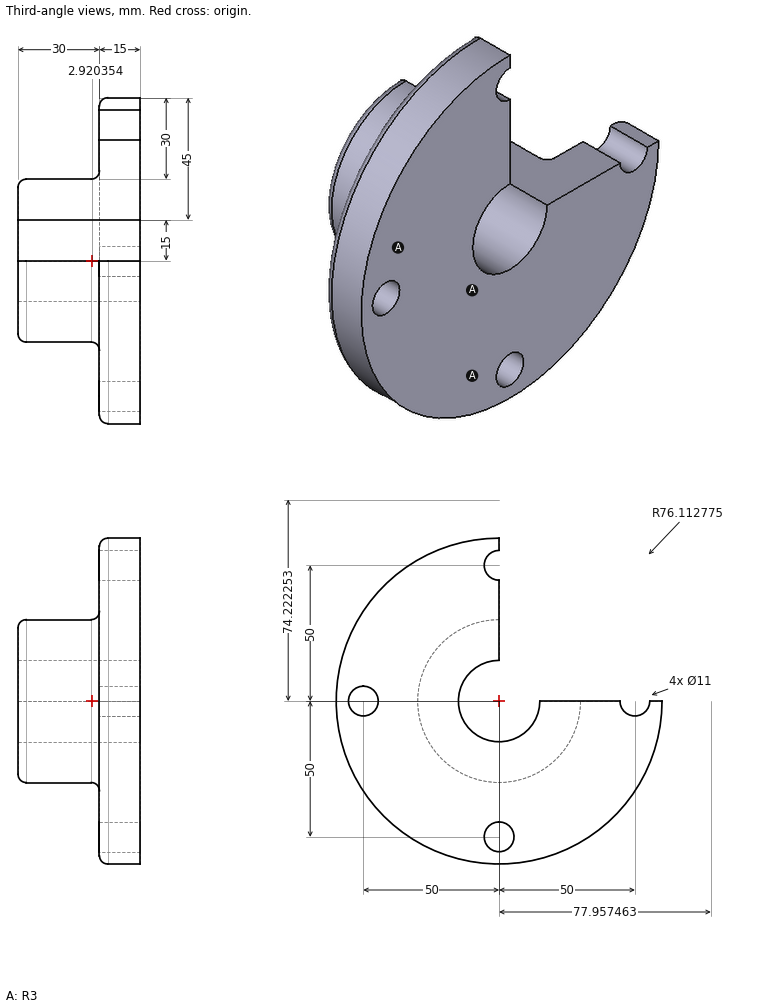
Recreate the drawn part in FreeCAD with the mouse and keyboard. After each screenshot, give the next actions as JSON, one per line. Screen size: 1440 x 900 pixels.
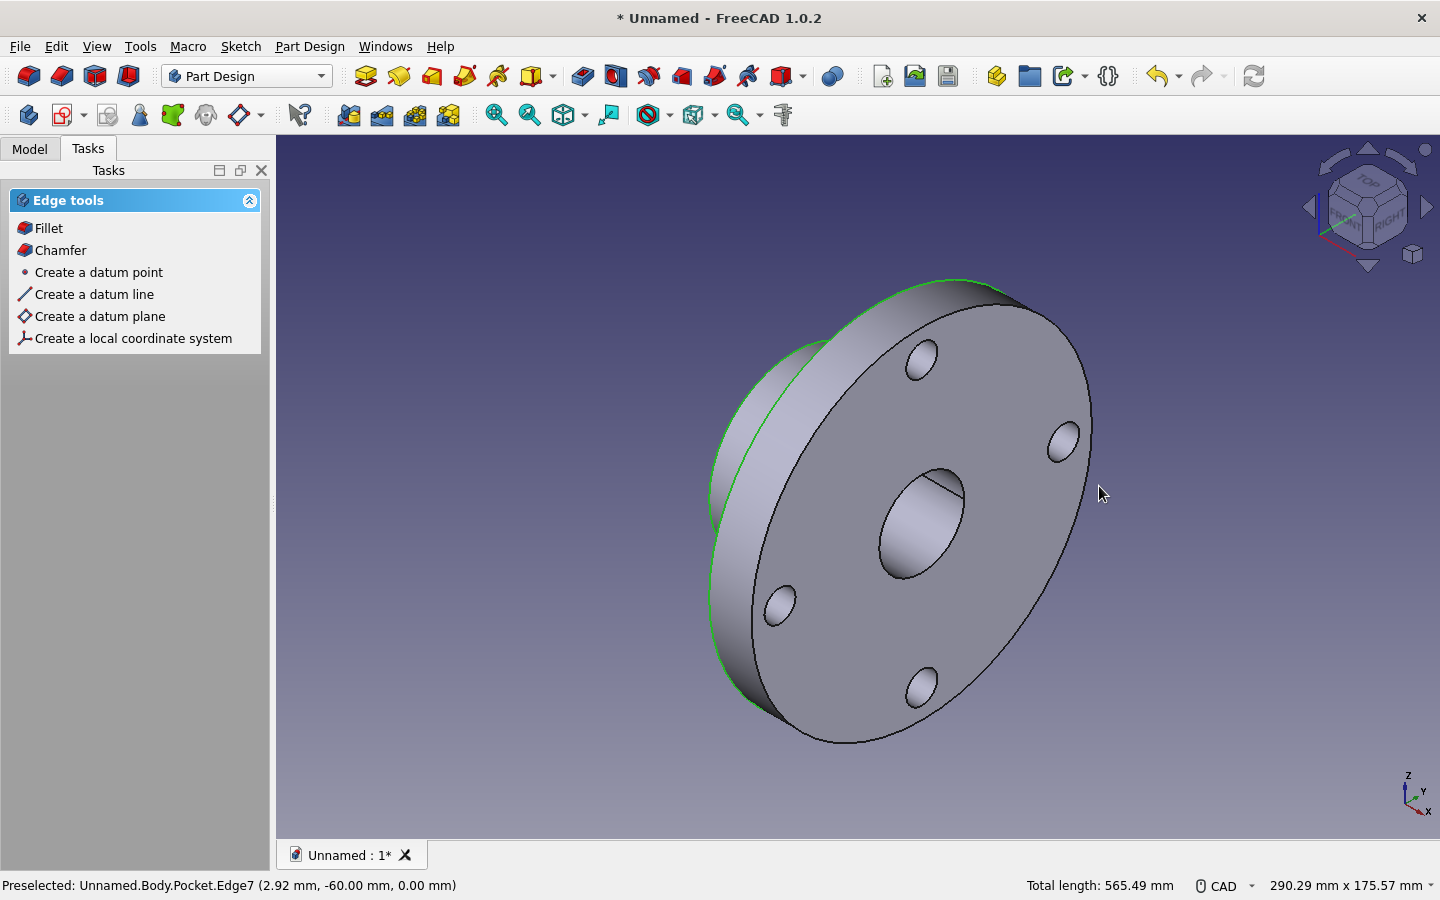
{"action": "key", "text": "2"}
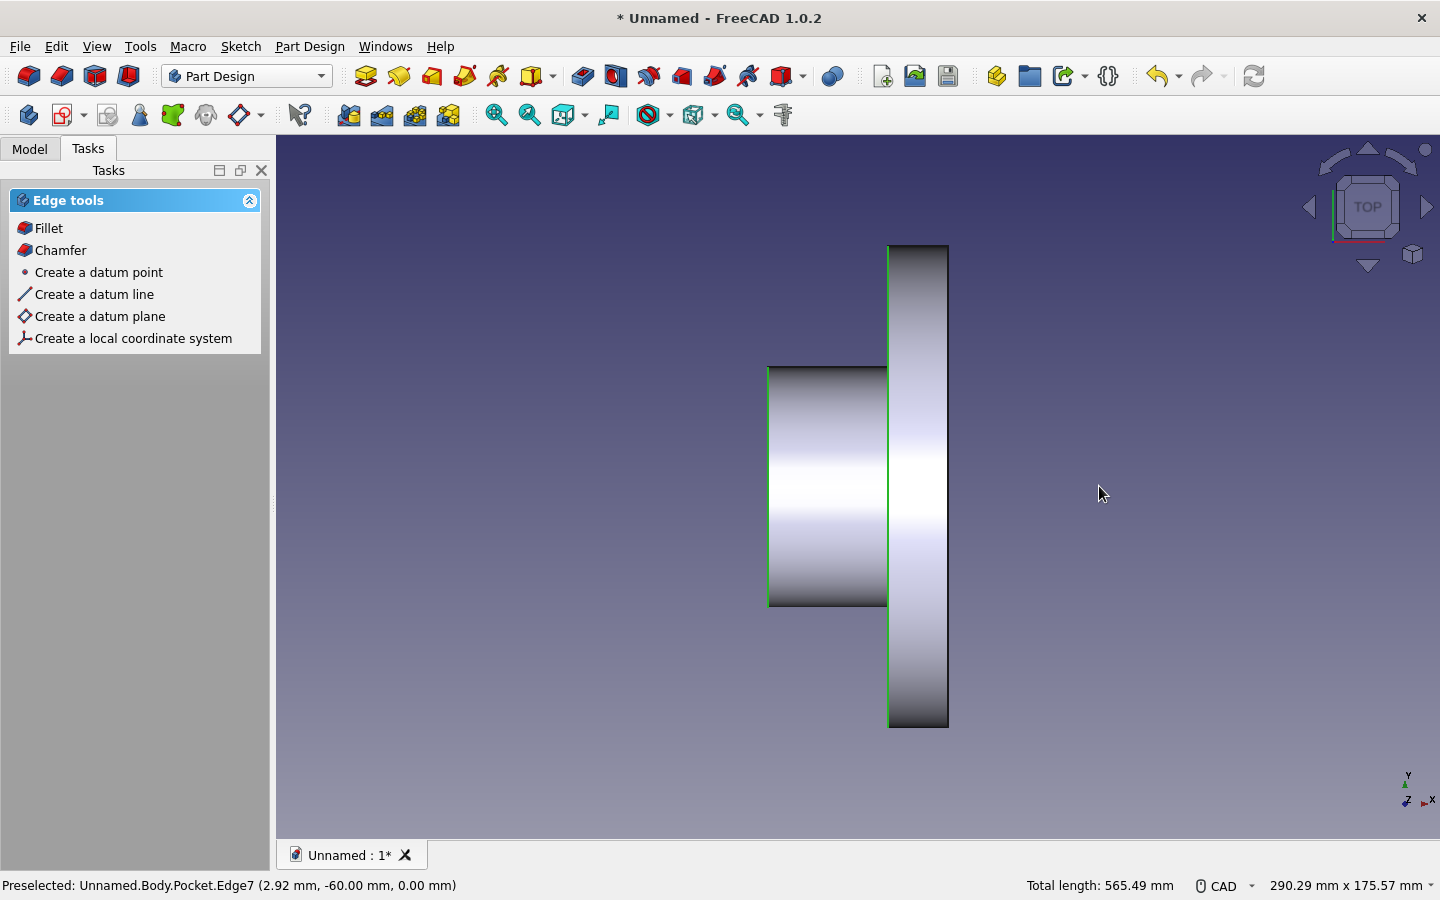
{"action": "key", "text": "1"}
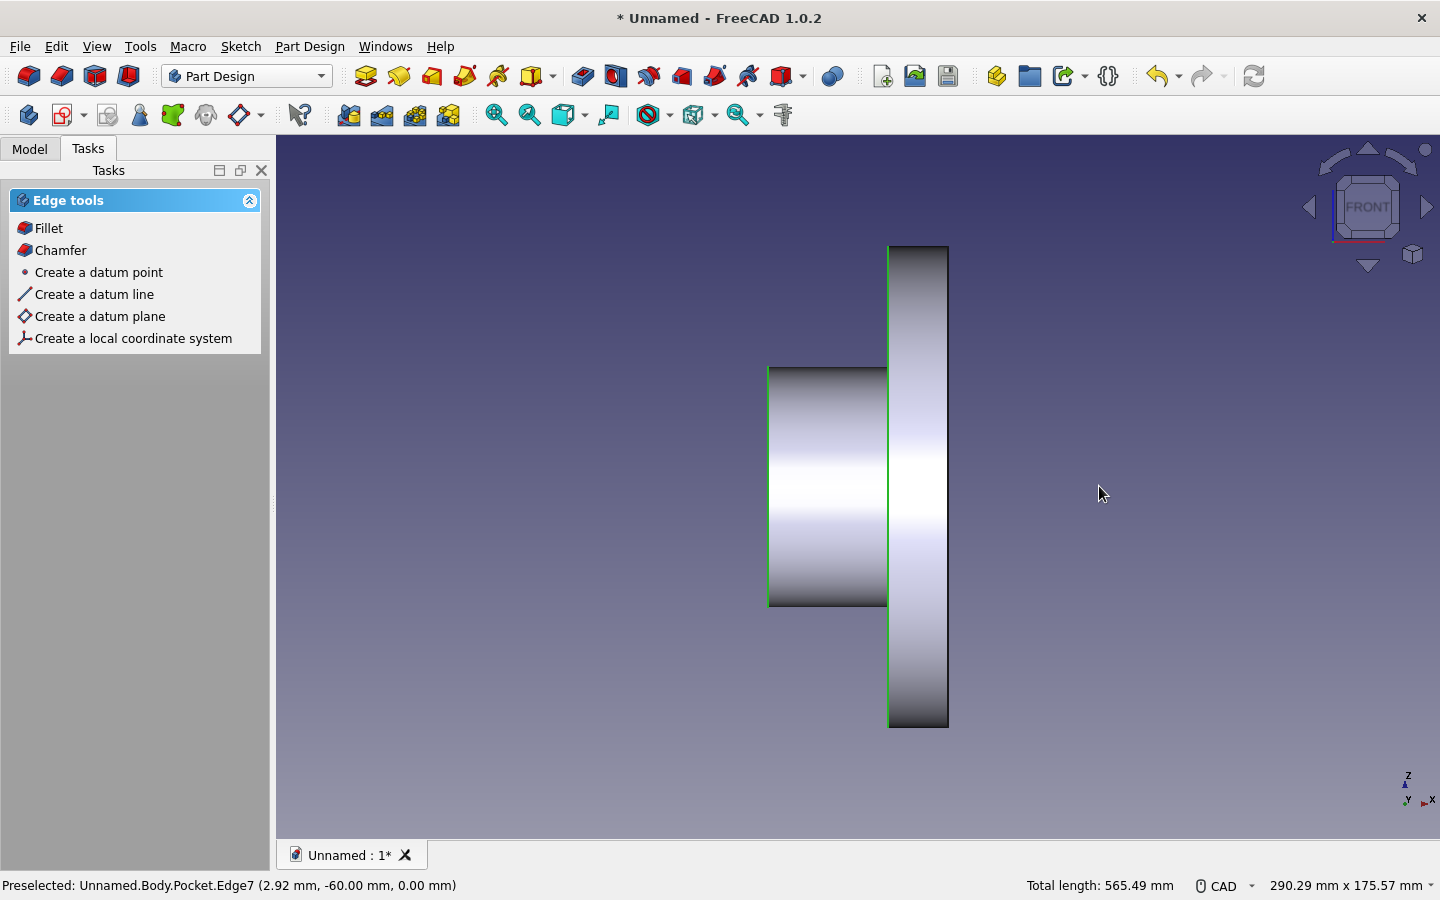
{"action": "key", "text": "3"}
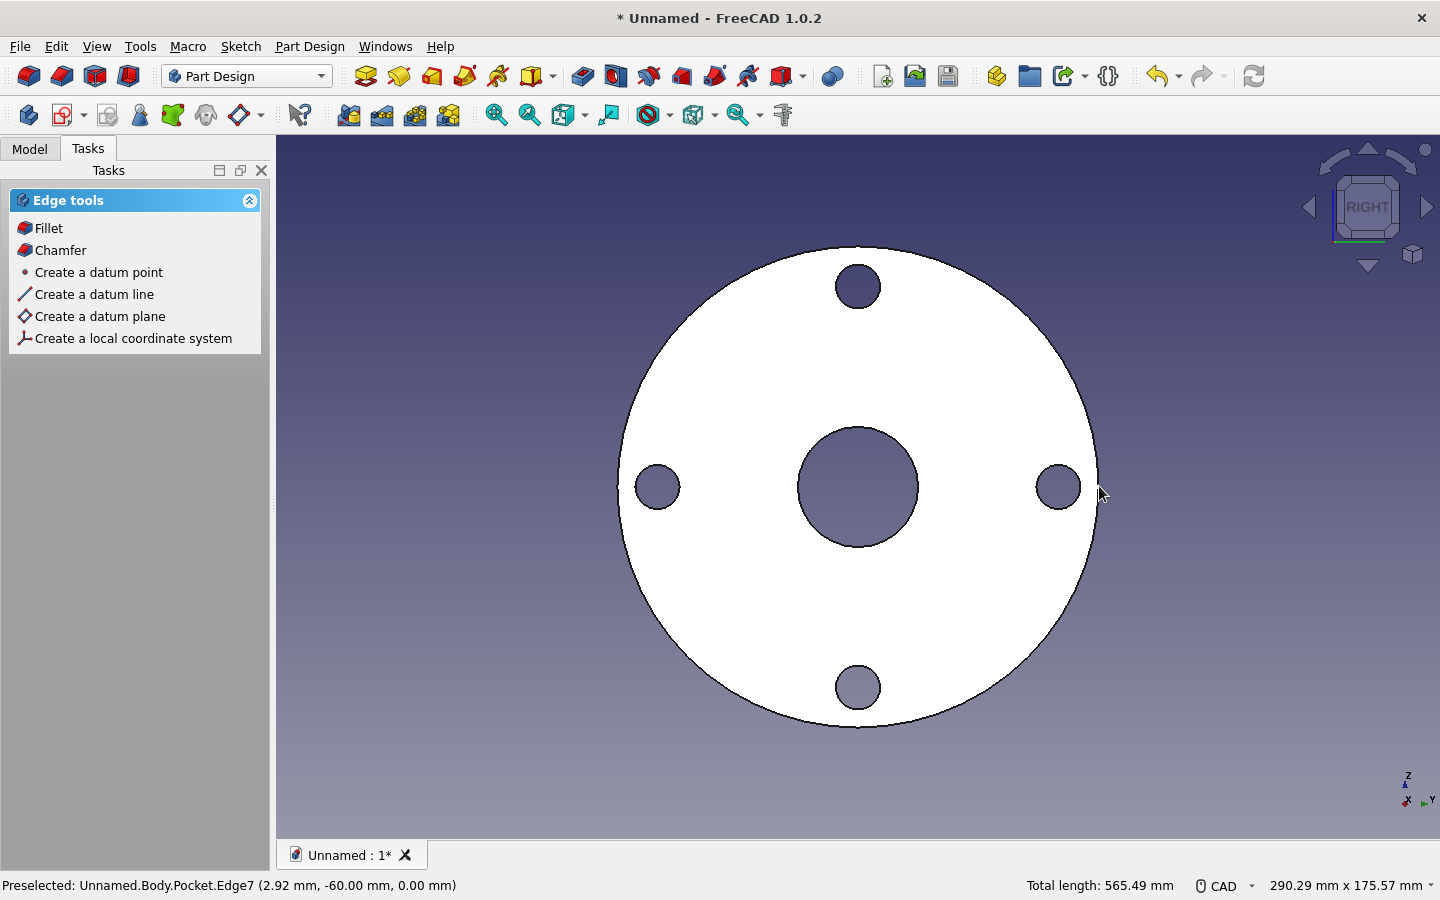
{"action": "key", "text": "5"}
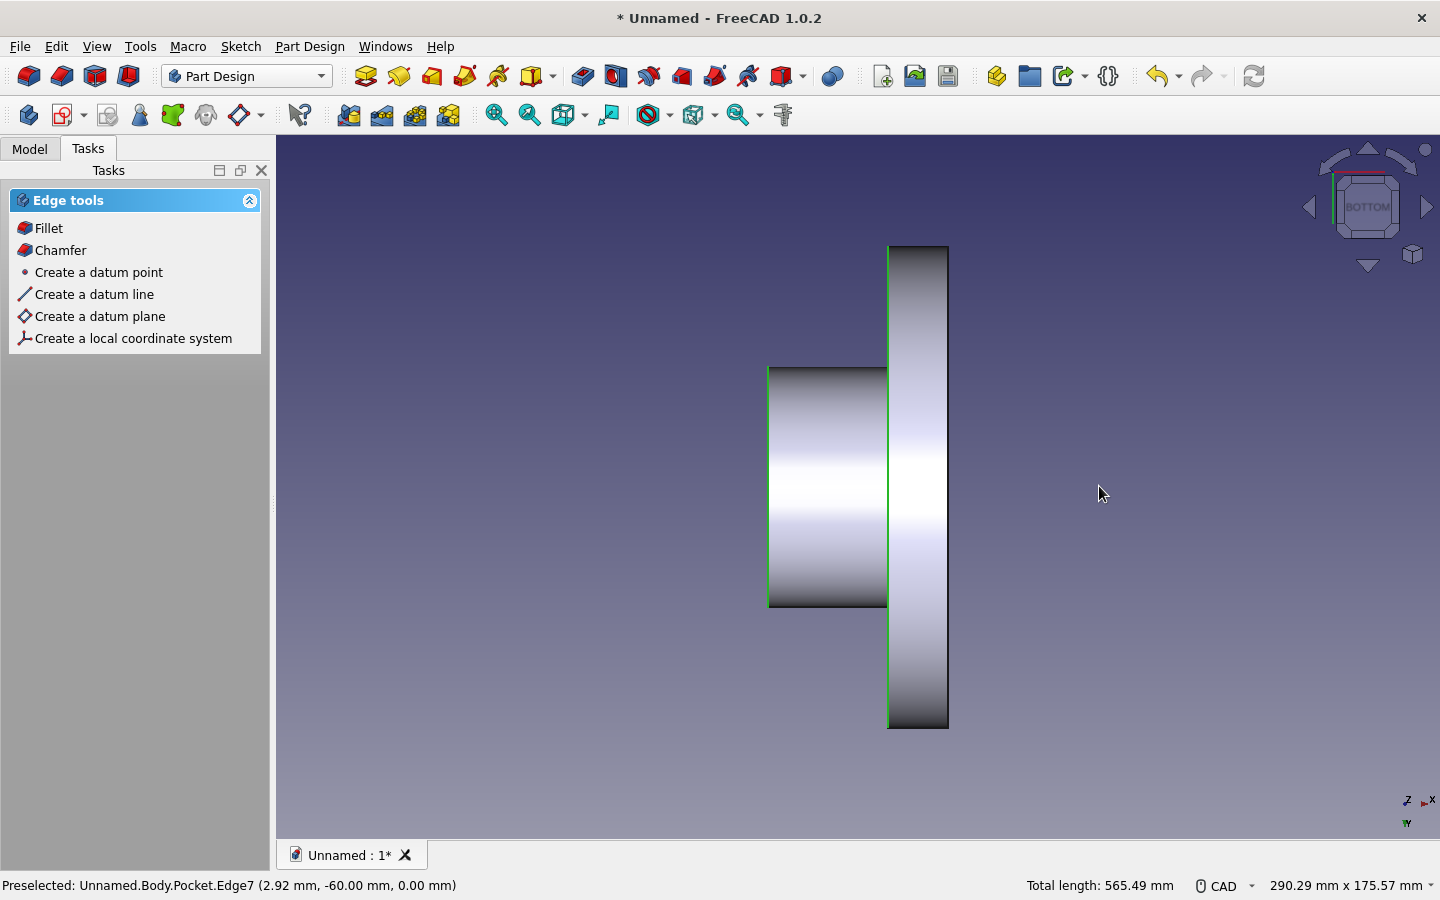
{"action": "key", "text": "4"}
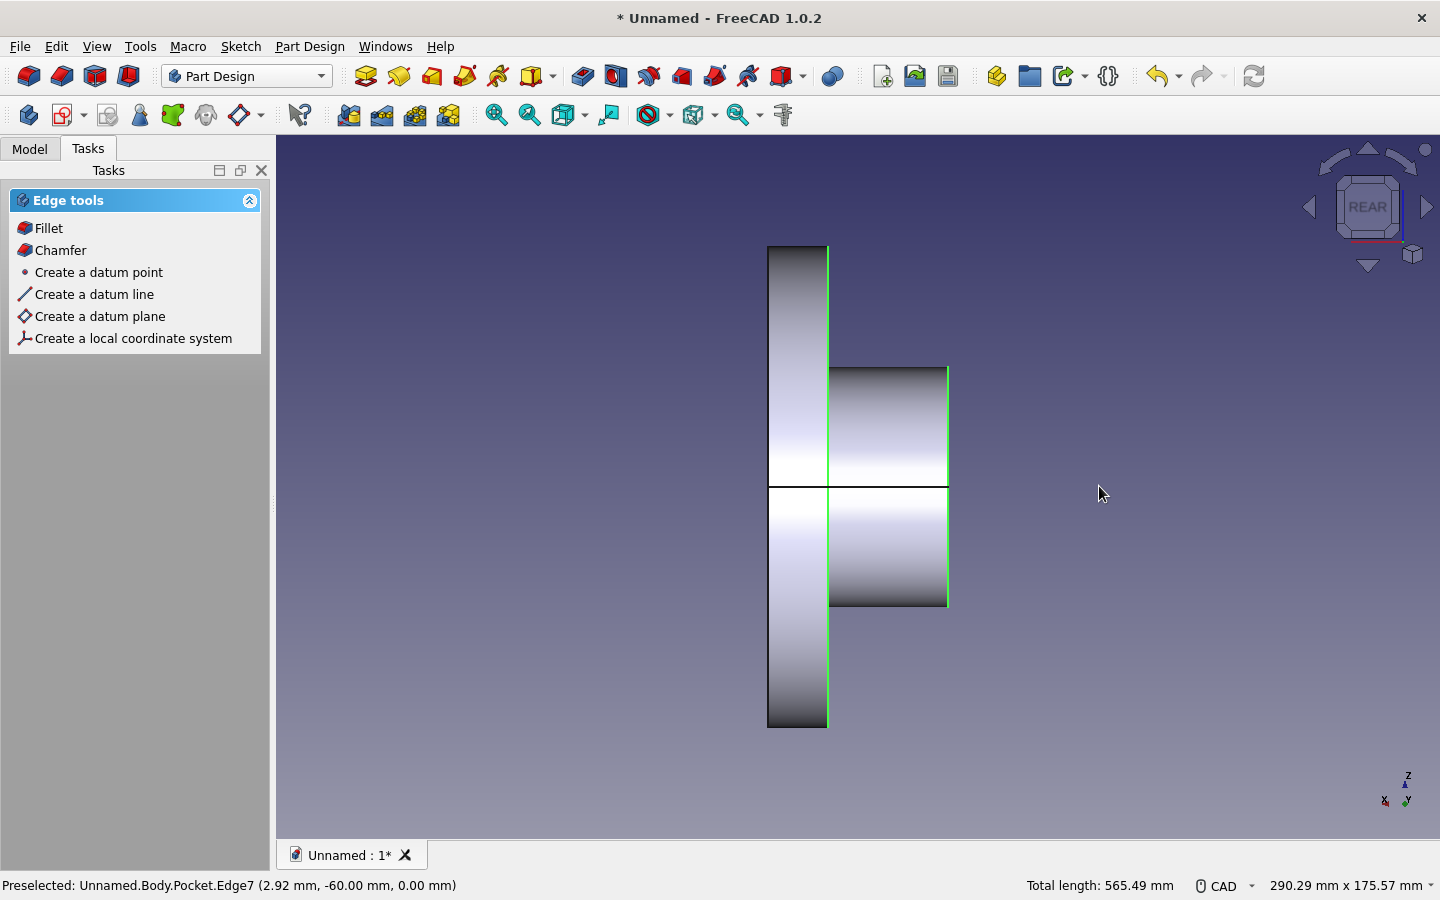
{"action": "key", "text": "6"}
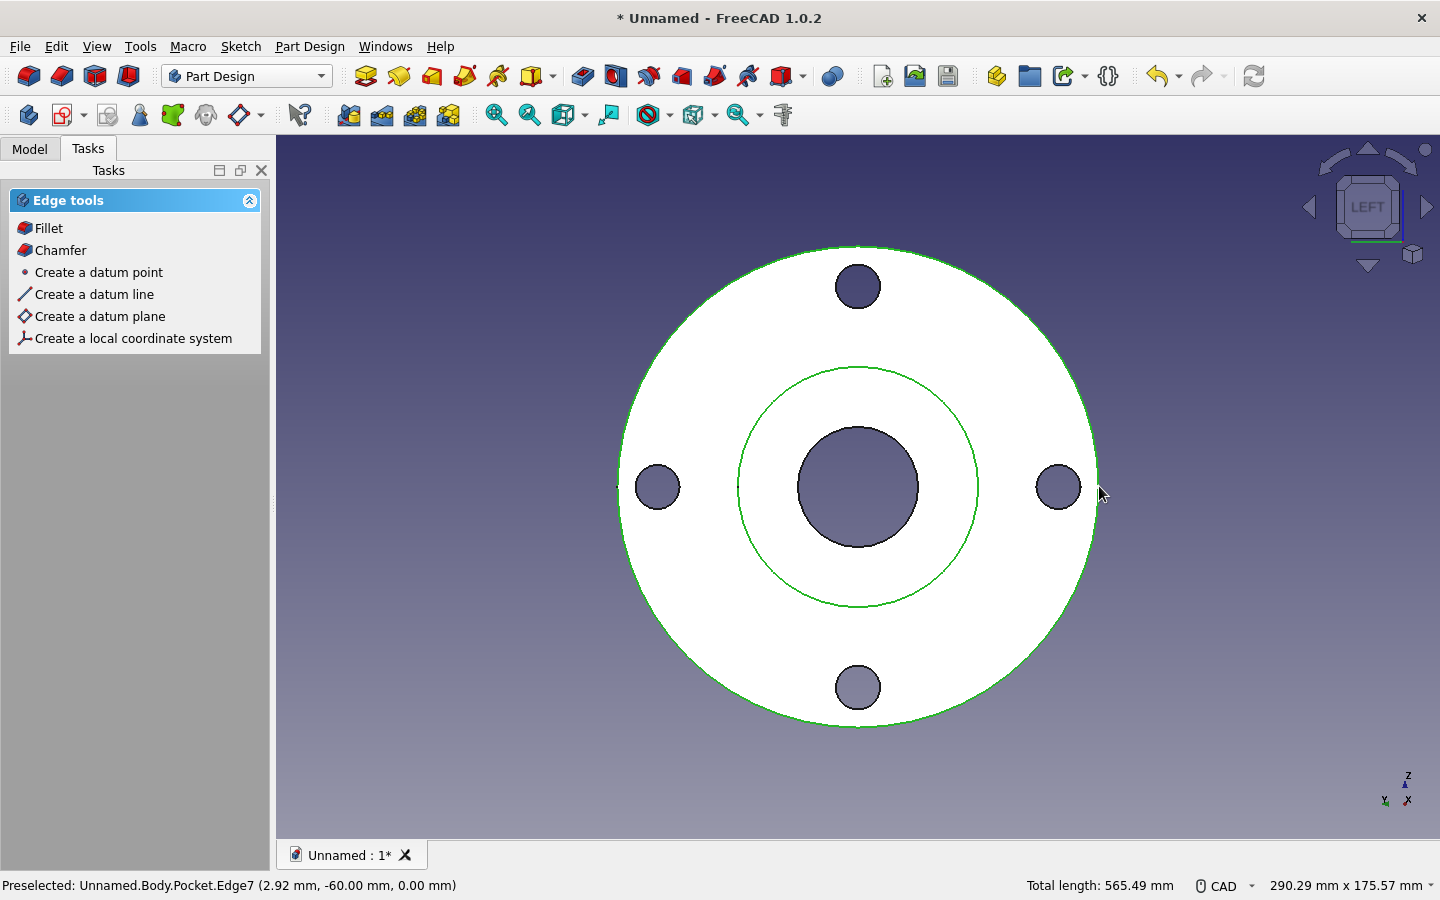
{"action": "key", "text": "v 3"}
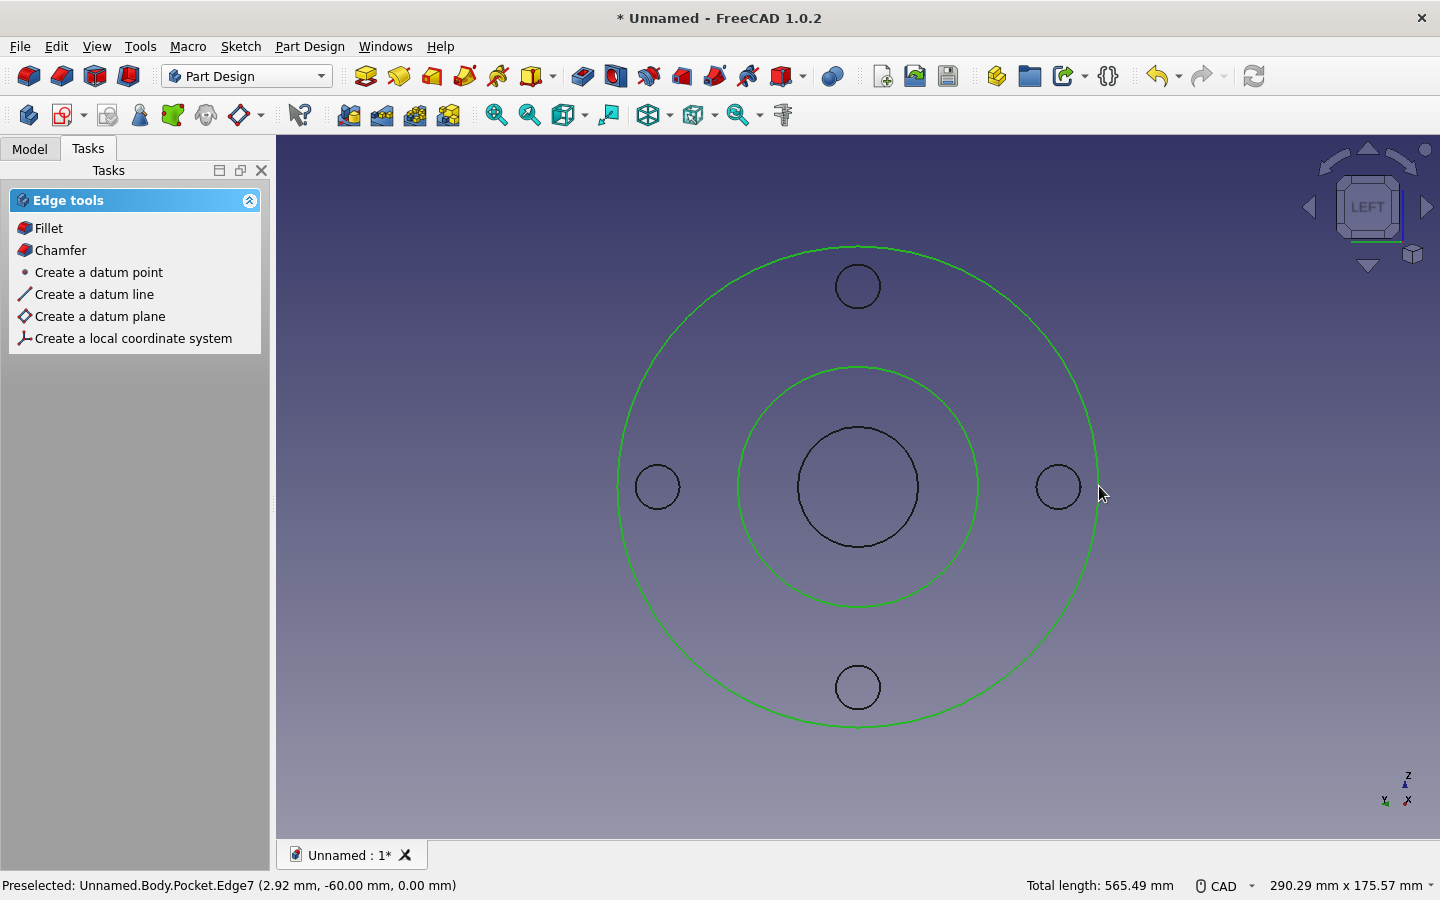
{"action": "key", "text": "0"}